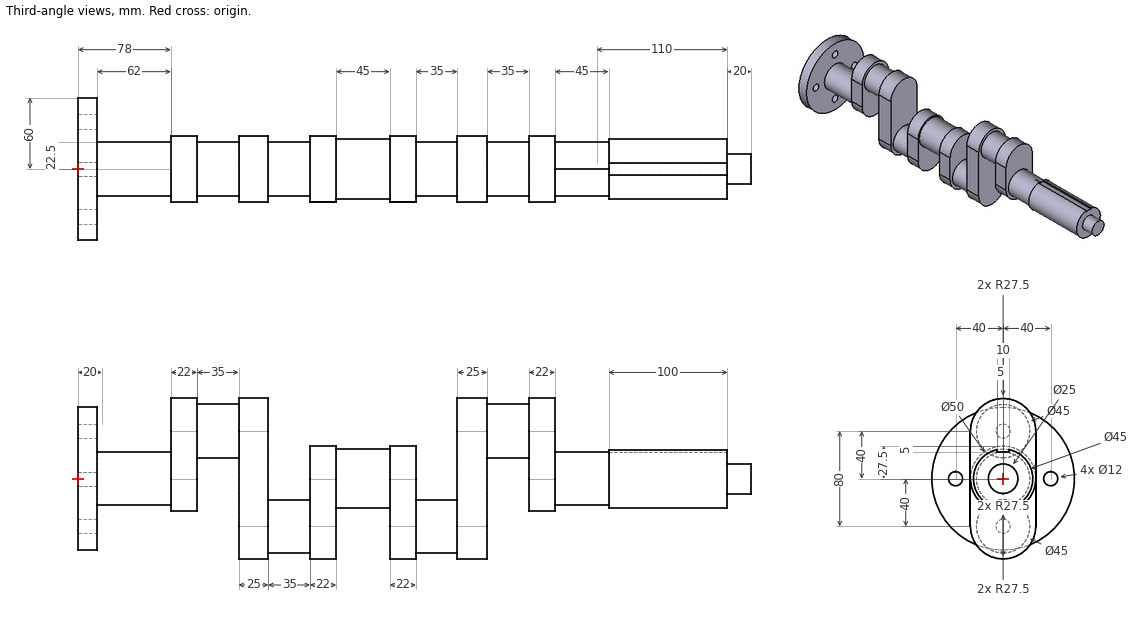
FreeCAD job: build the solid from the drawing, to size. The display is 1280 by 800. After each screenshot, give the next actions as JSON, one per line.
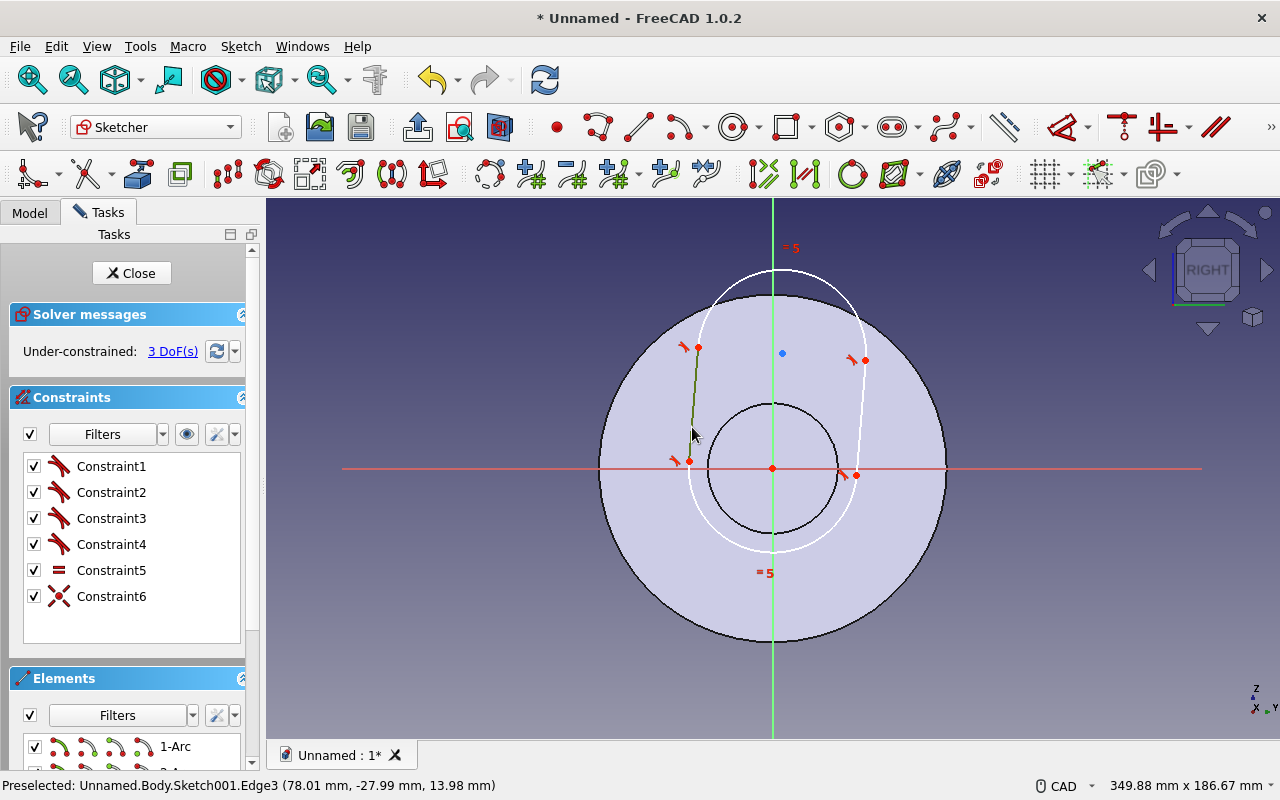
{"action": "left_click", "coordinate": [1188, 128]}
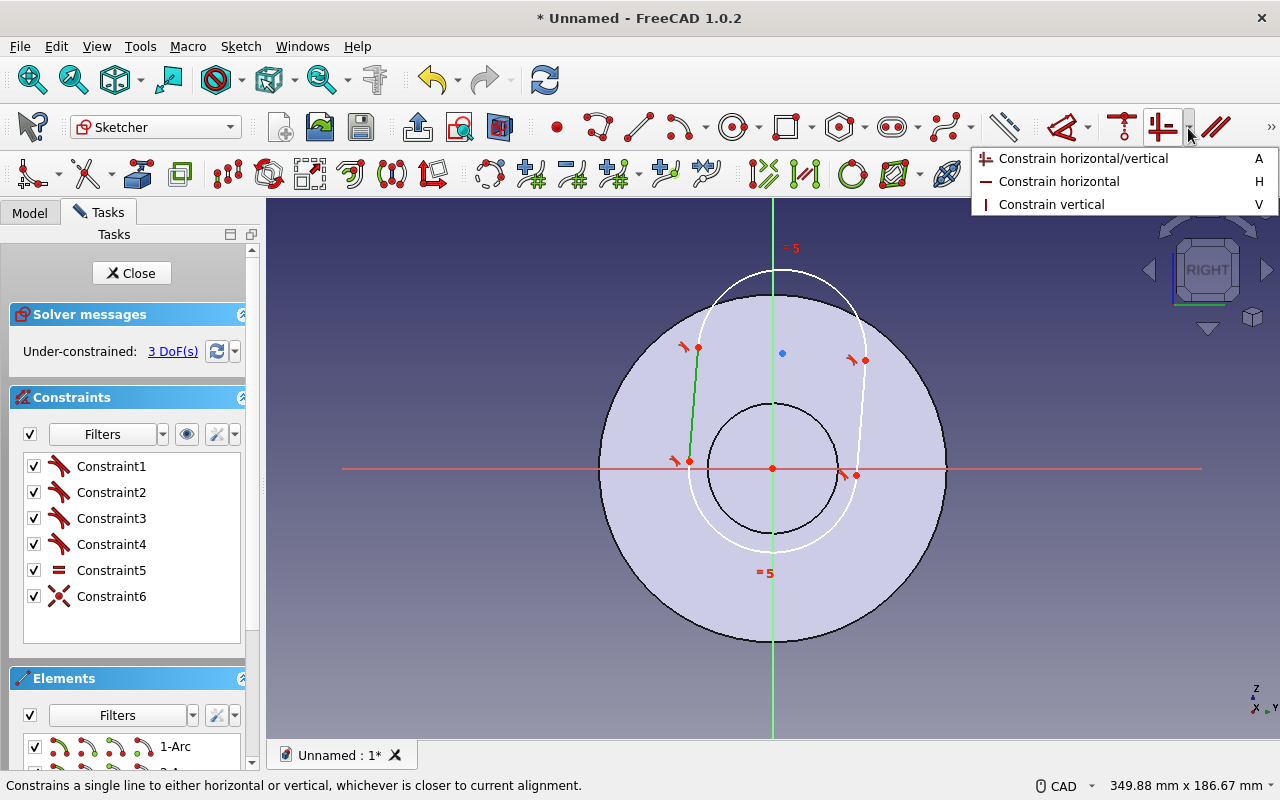
{"action": "left_click", "coordinate": [1125, 204]}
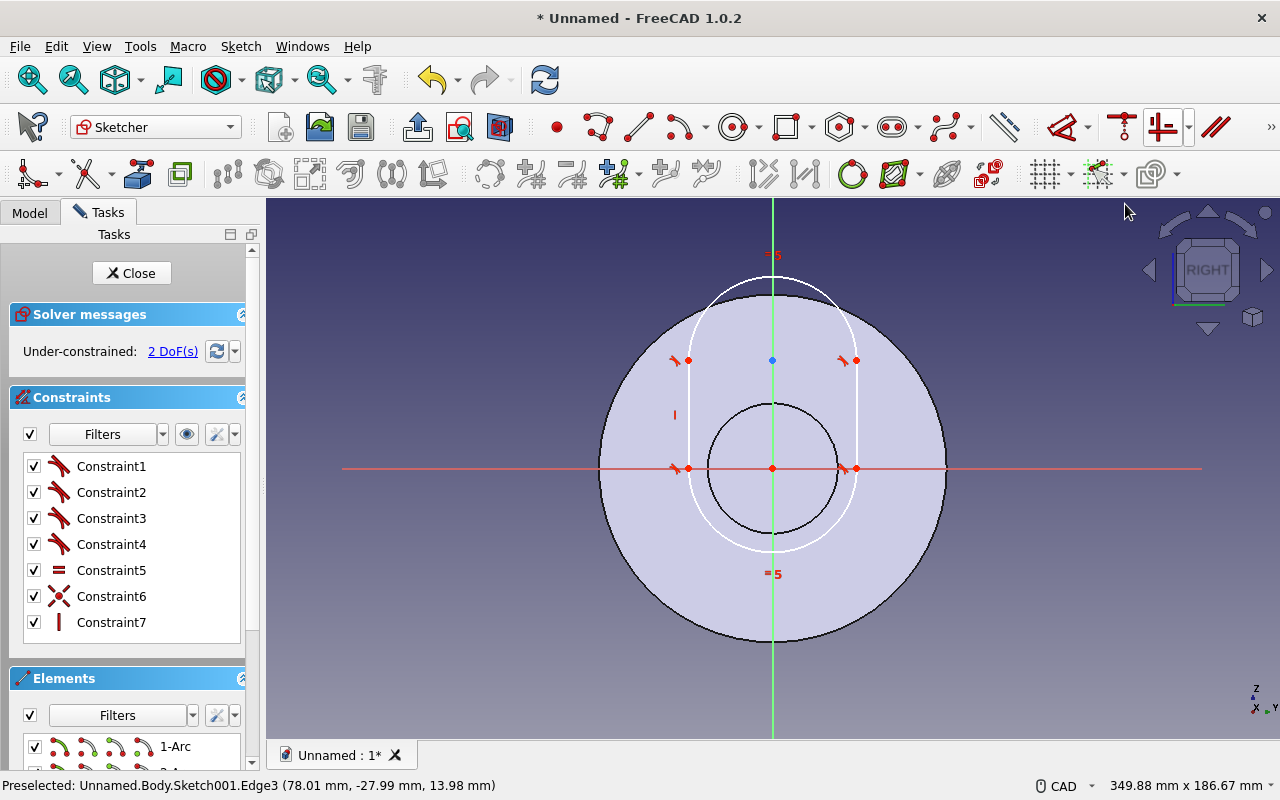
{"action": "key", "text": "d"}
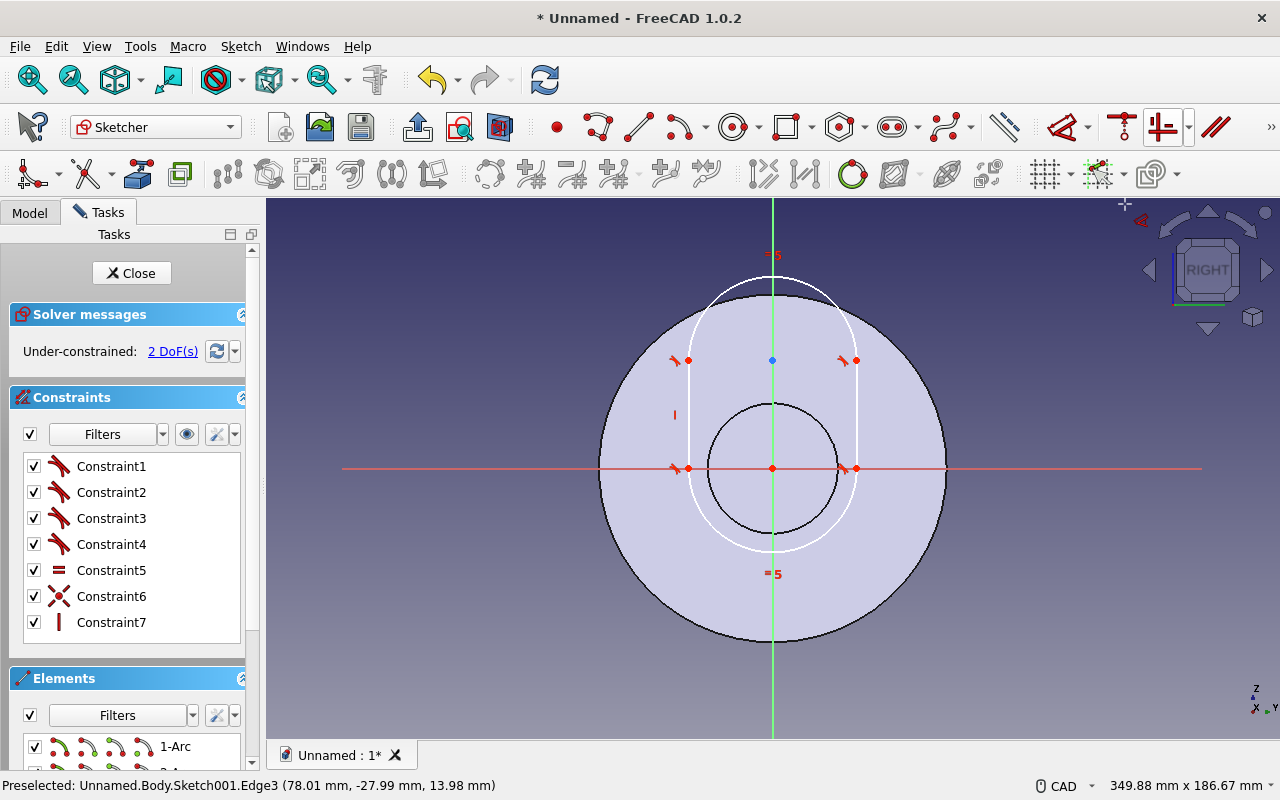
{"action": "left_click", "coordinate": [724, 536]}
{"action": "left_click", "coordinate": [705, 562]}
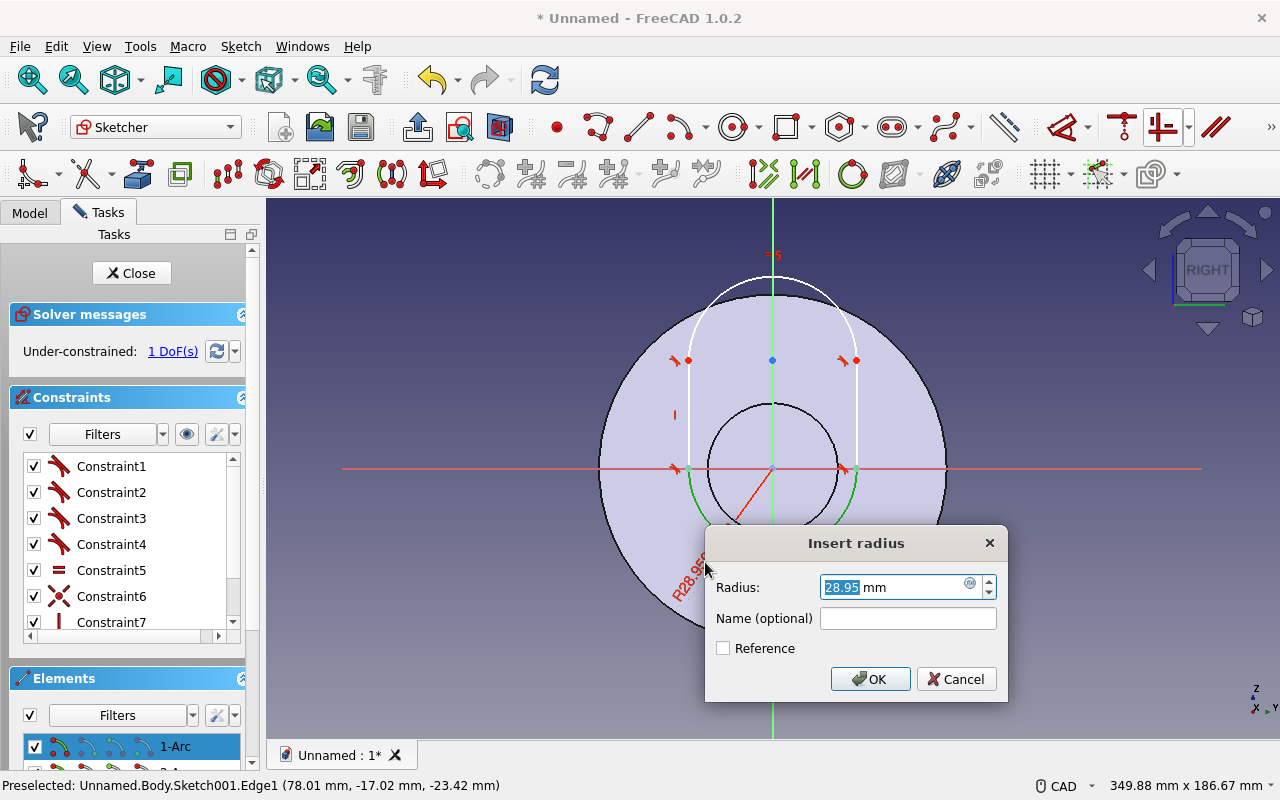
{"action": "type", "text": "27.5"}
{"action": "key", "text": "Return"}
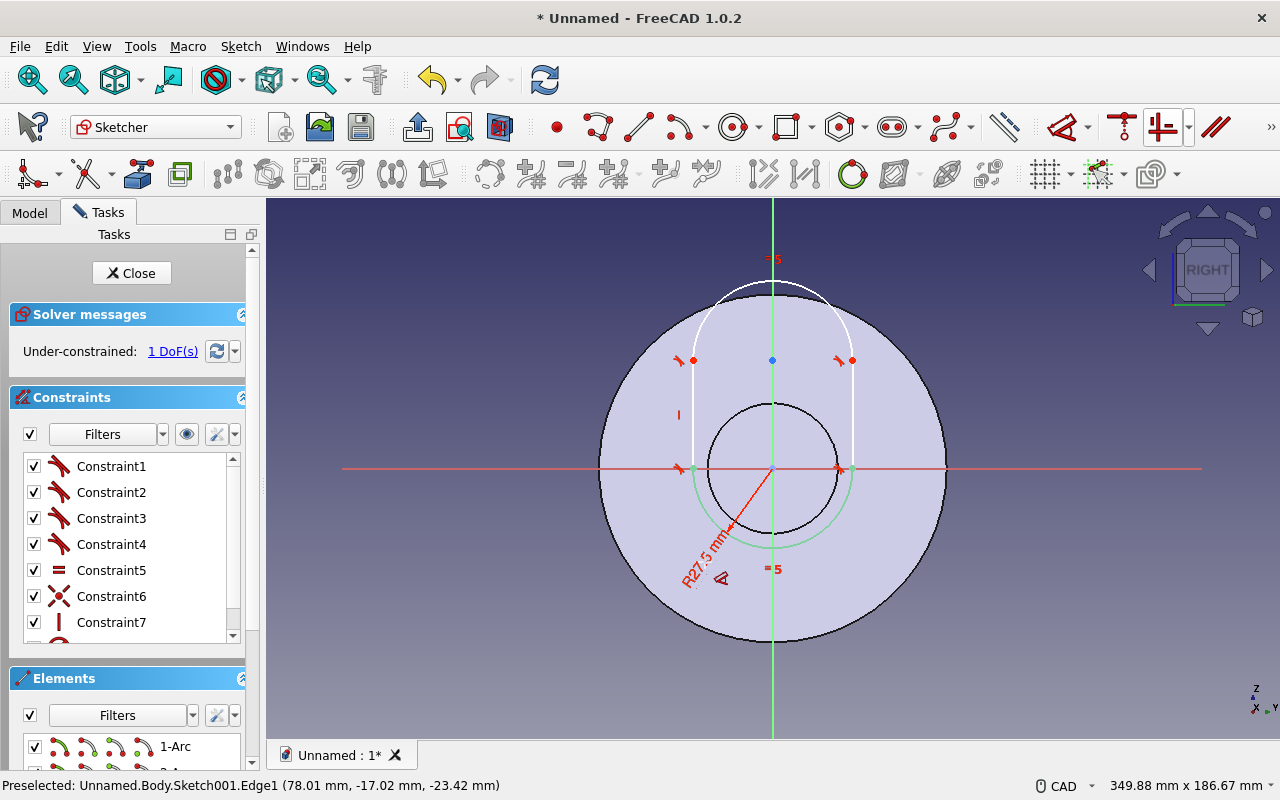
{"action": "left_click", "coordinate": [693, 436]}
{"action": "left_click", "coordinate": [659, 415]}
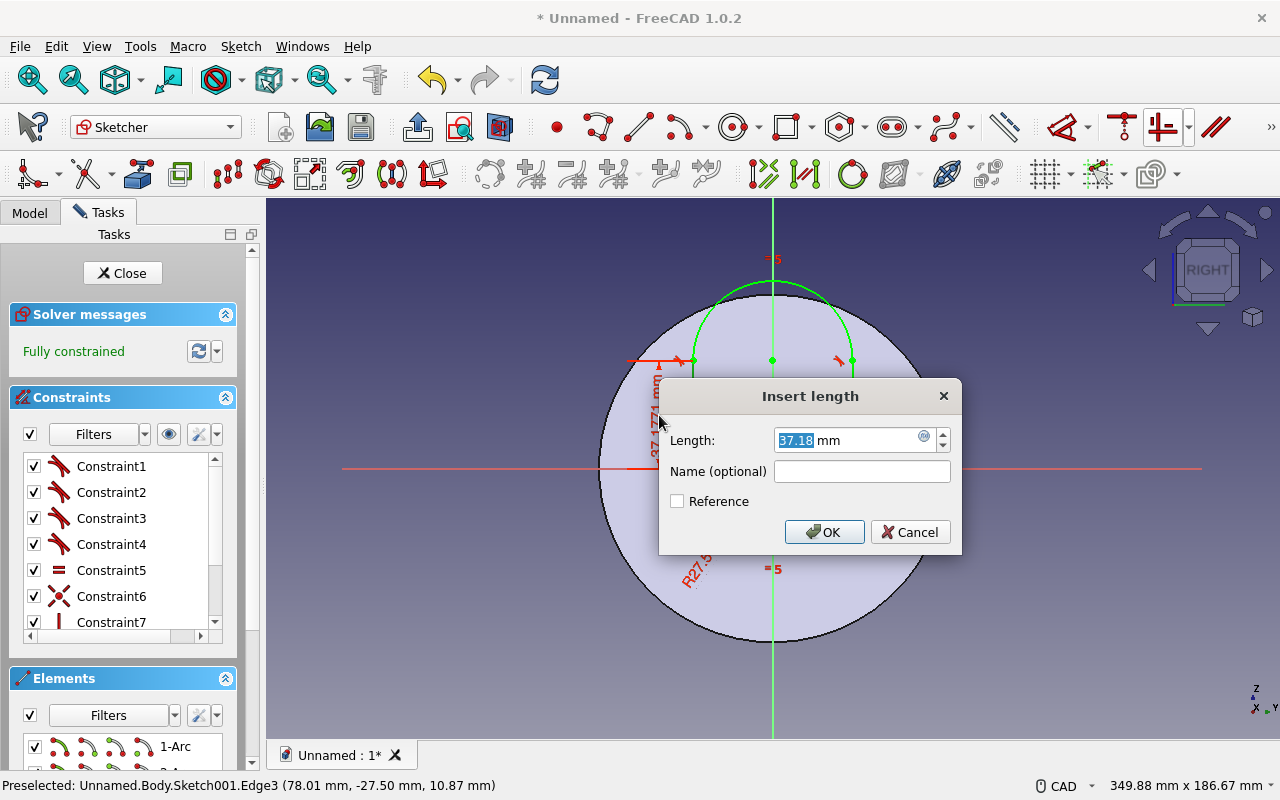
{"action": "type", "text": "40"}
{"action": "key", "text": "Return"}
{"action": "key", "text": "Escape"}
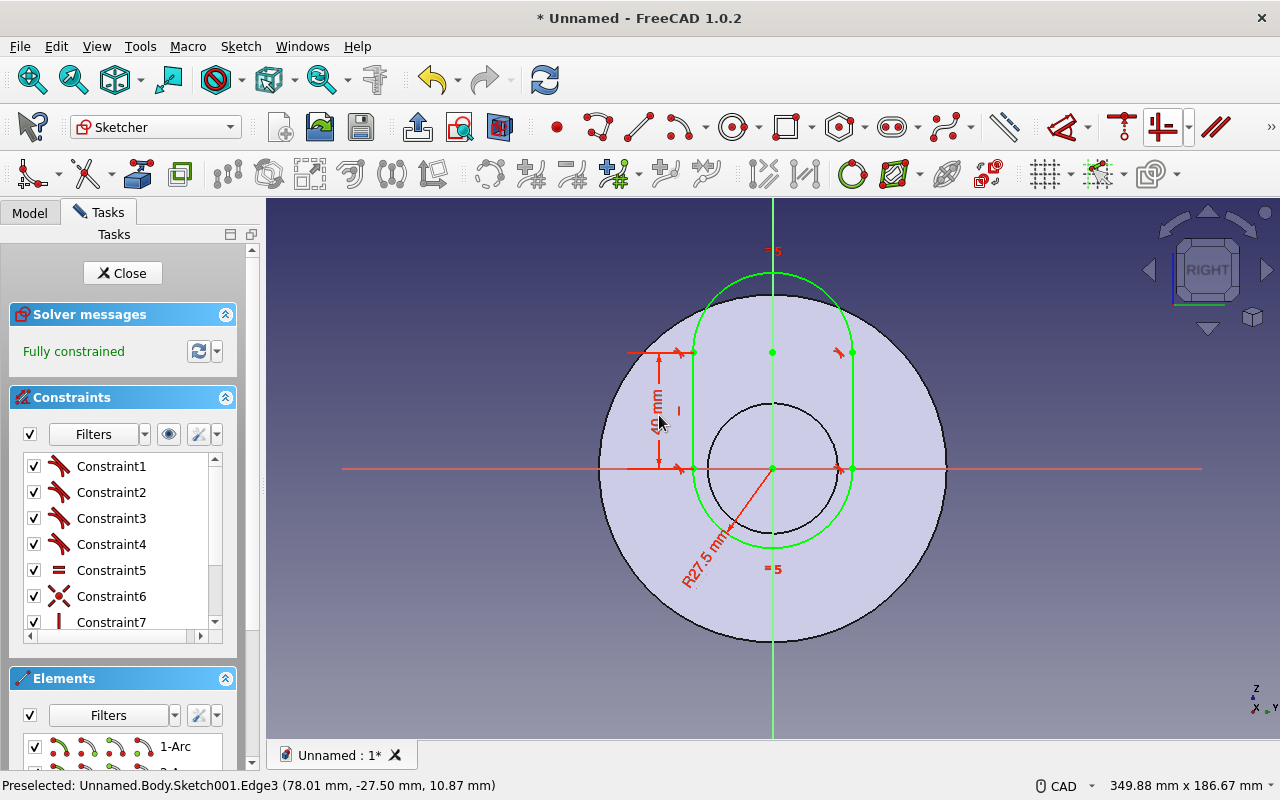
{"action": "left_click", "coordinate": [123, 273]}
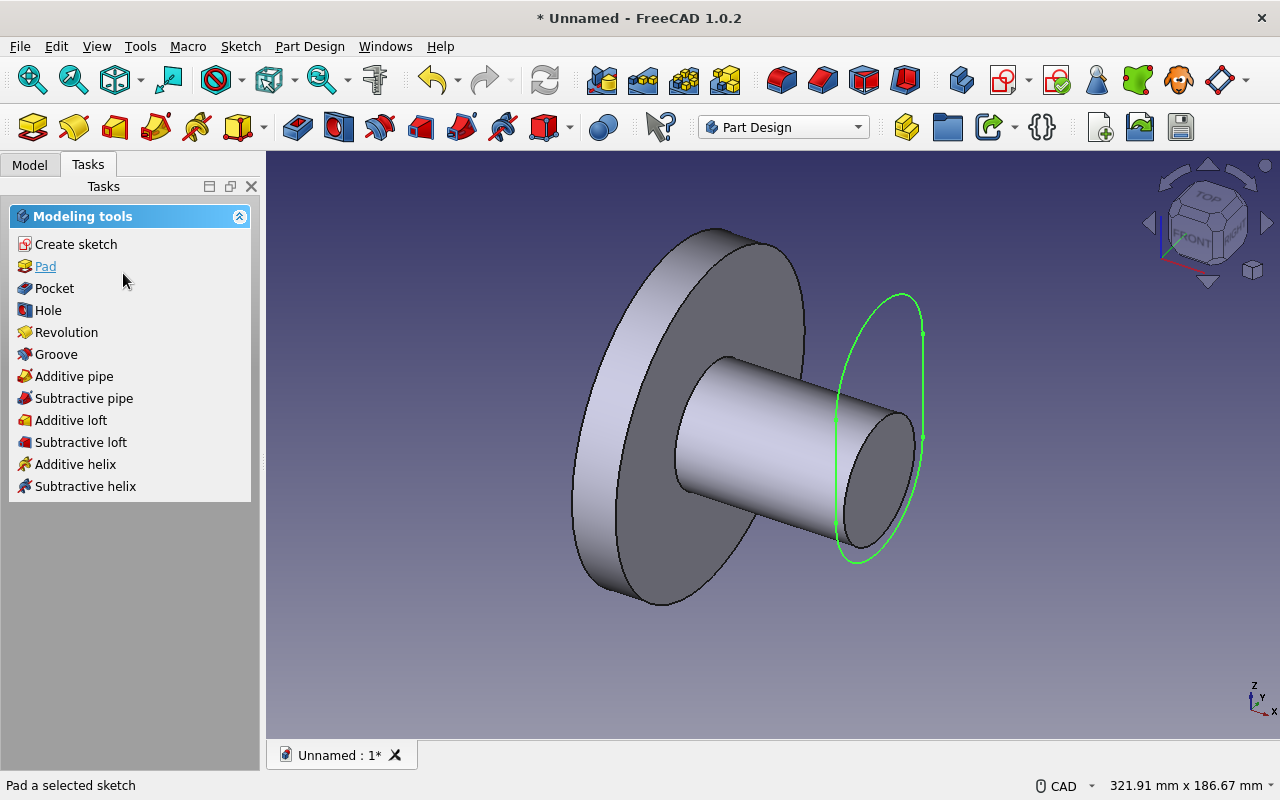
{"action": "left_click", "coordinate": [33, 128]}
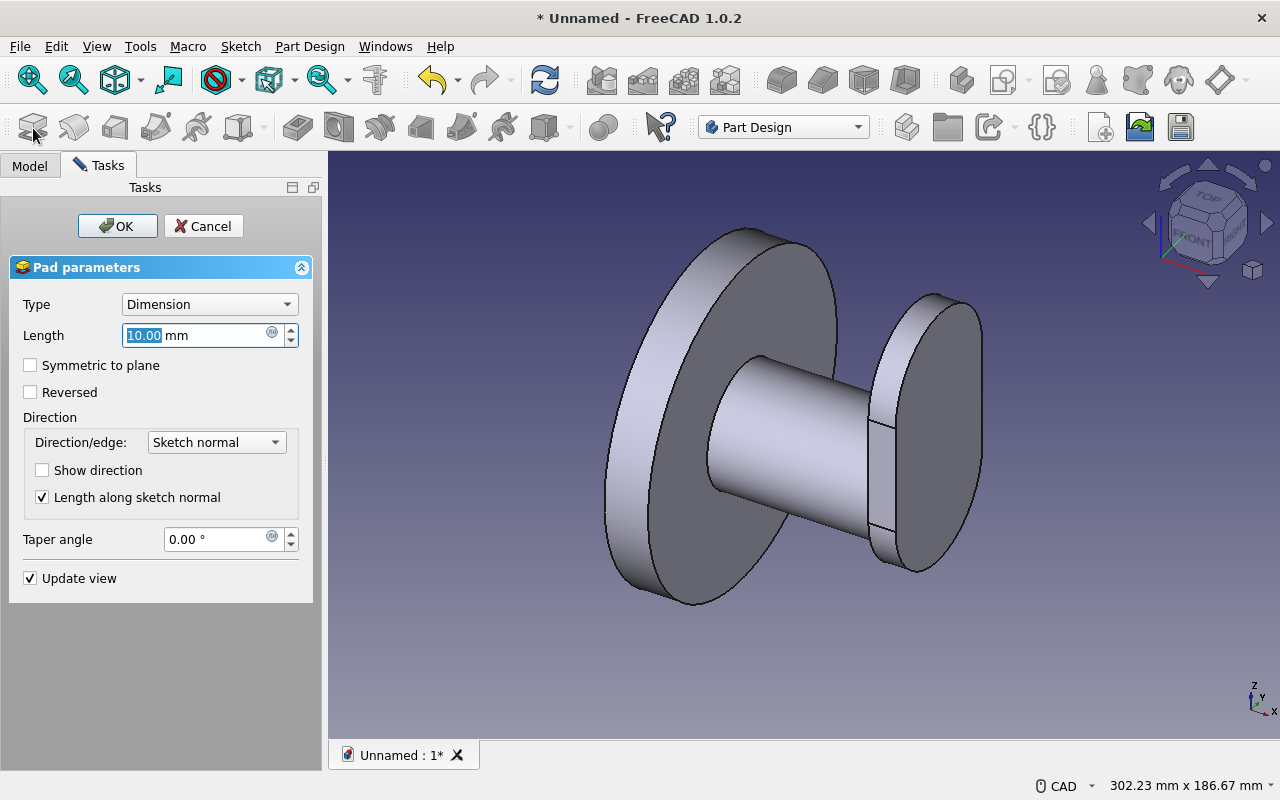
{"action": "type", "text": "22"}
{"action": "key", "text": "Tab"}